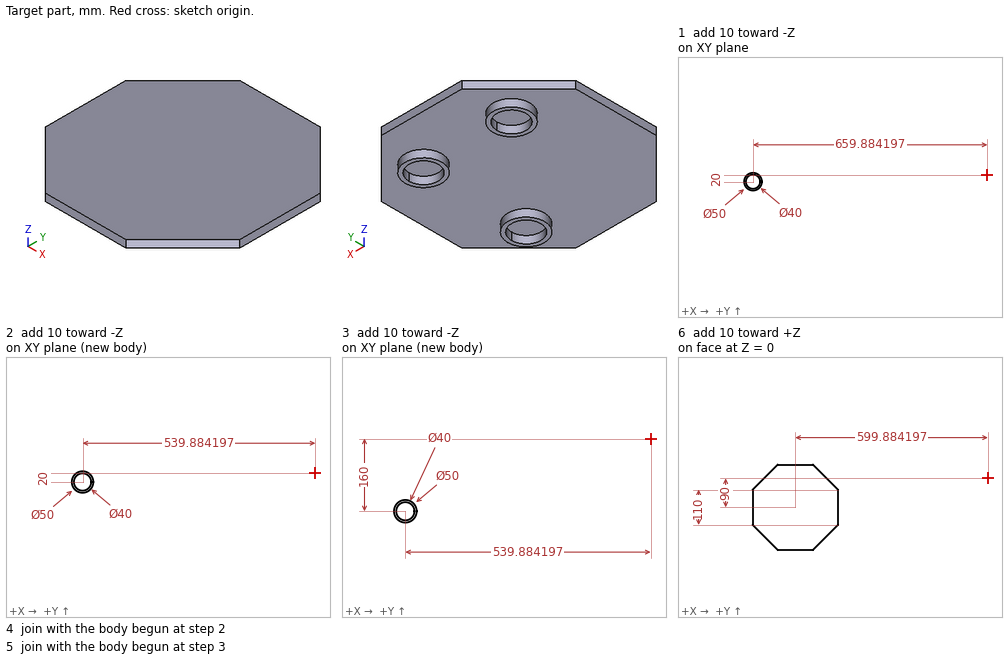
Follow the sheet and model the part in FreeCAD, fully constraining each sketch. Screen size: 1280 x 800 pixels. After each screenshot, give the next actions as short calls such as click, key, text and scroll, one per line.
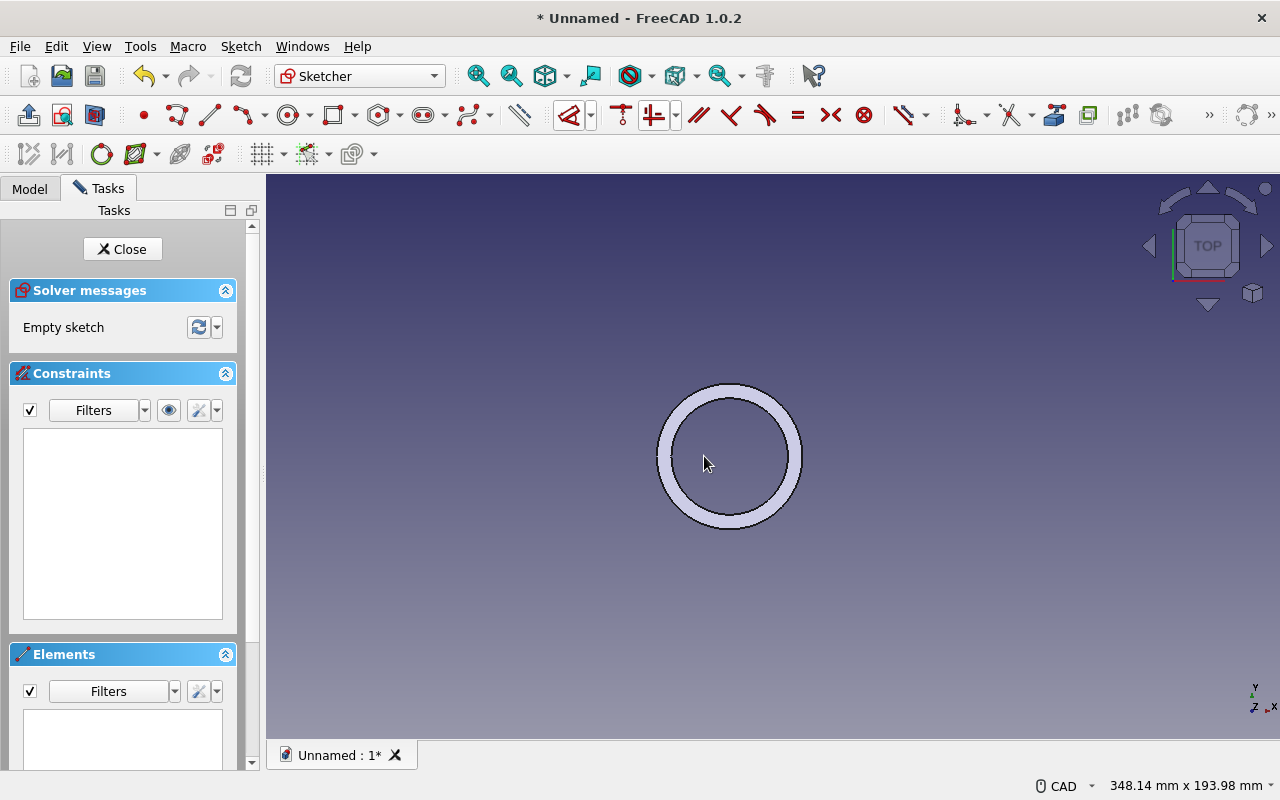
scroll(704, 456, down, 5)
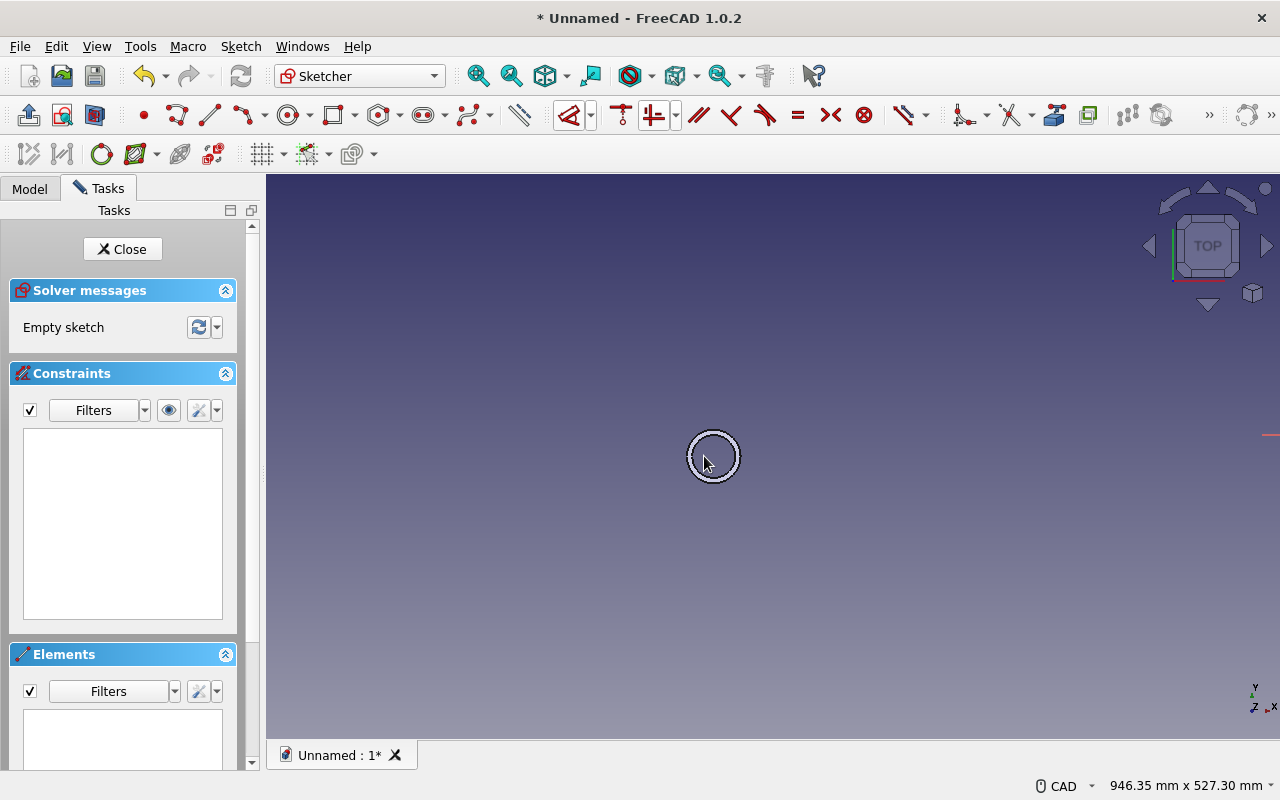
scroll(864, 456, up, 10)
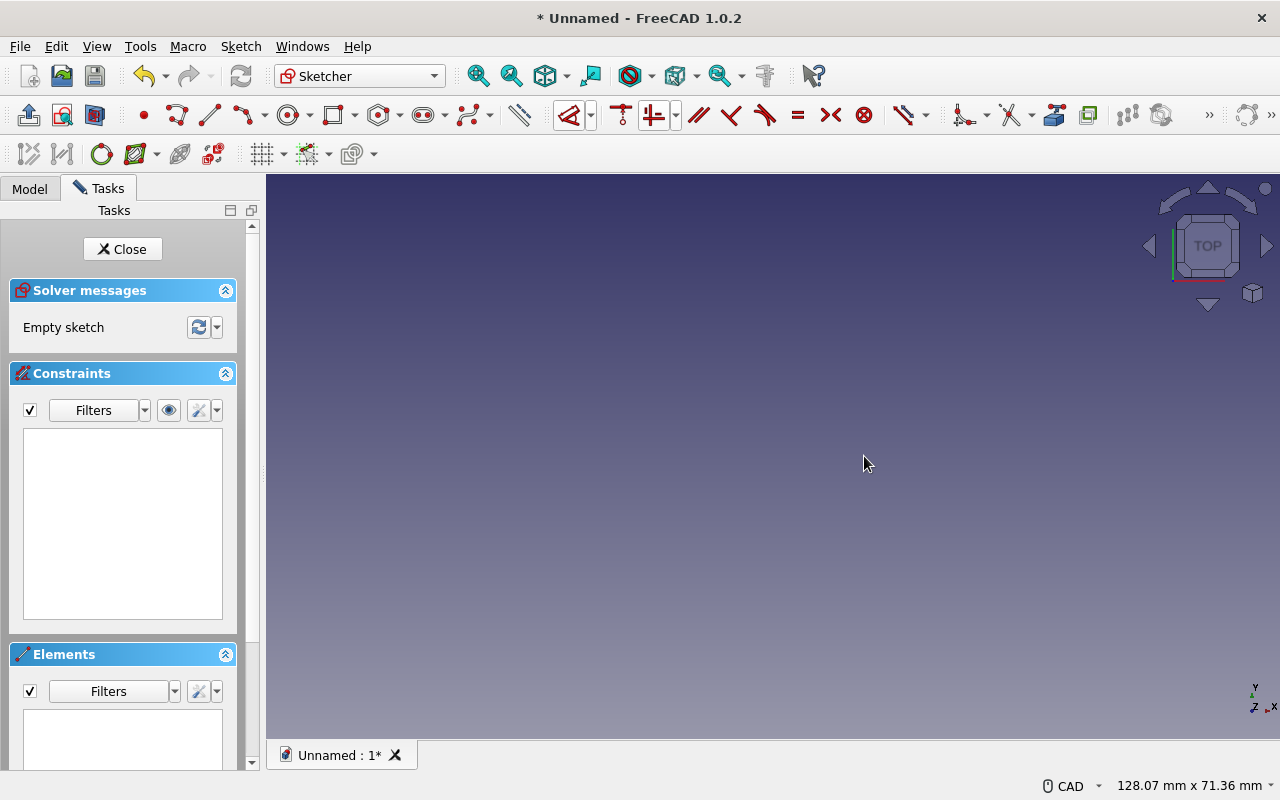
key(g)
key(c)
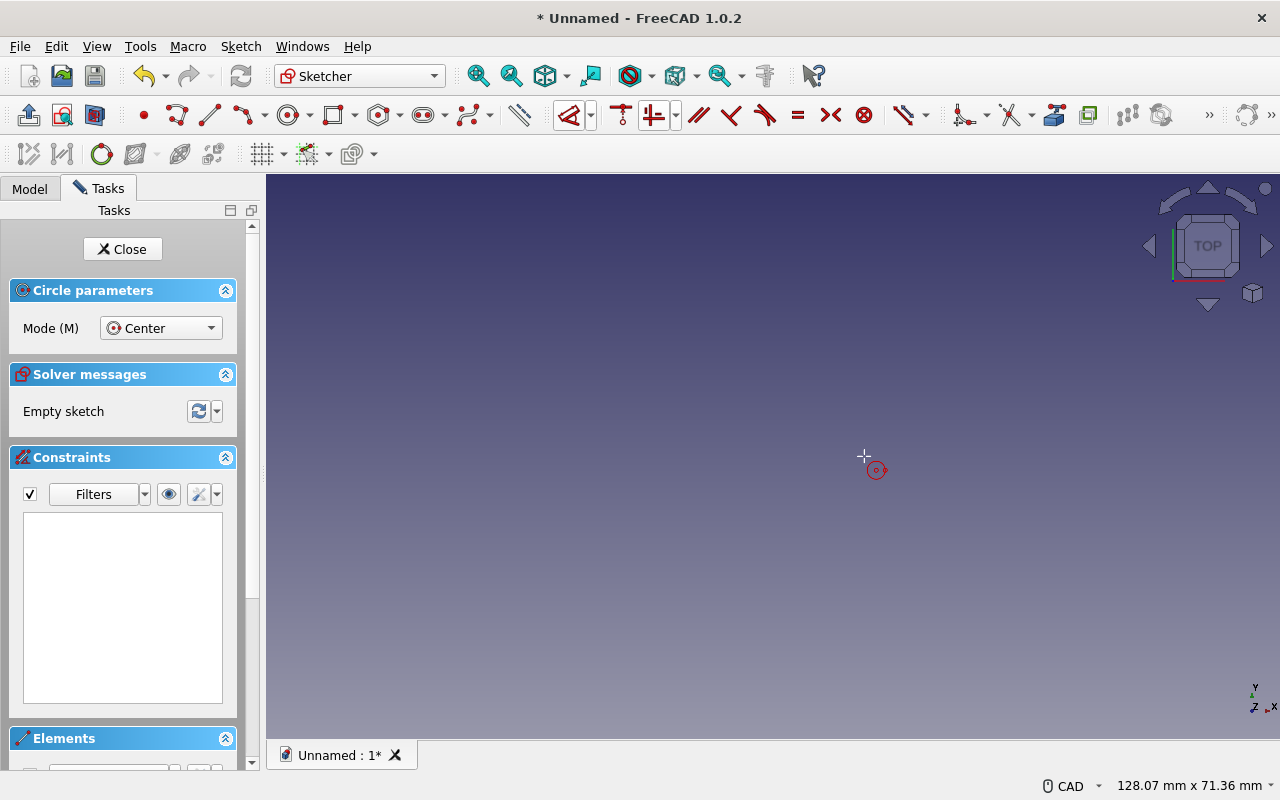
click(700, 456)
move(840, 317)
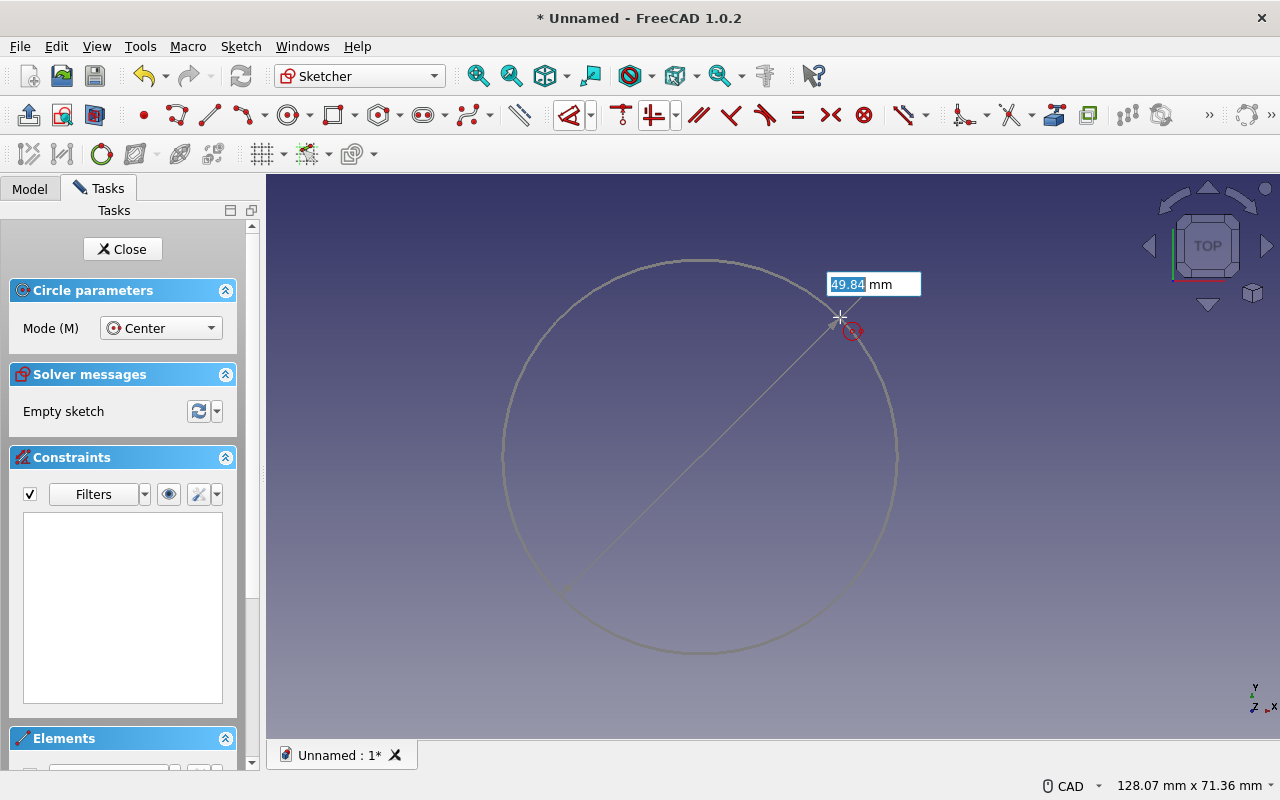
text(50)
key(Return)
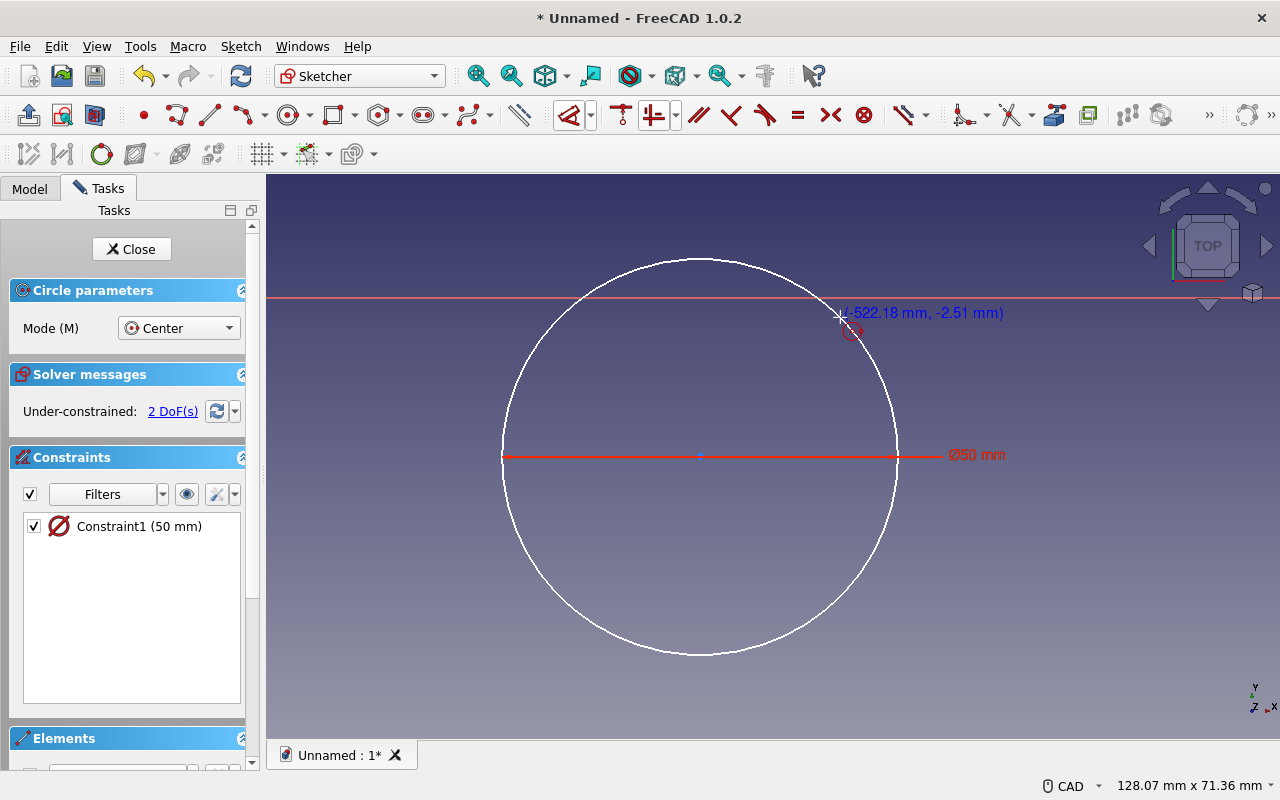
click(700, 457)
move(812, 345)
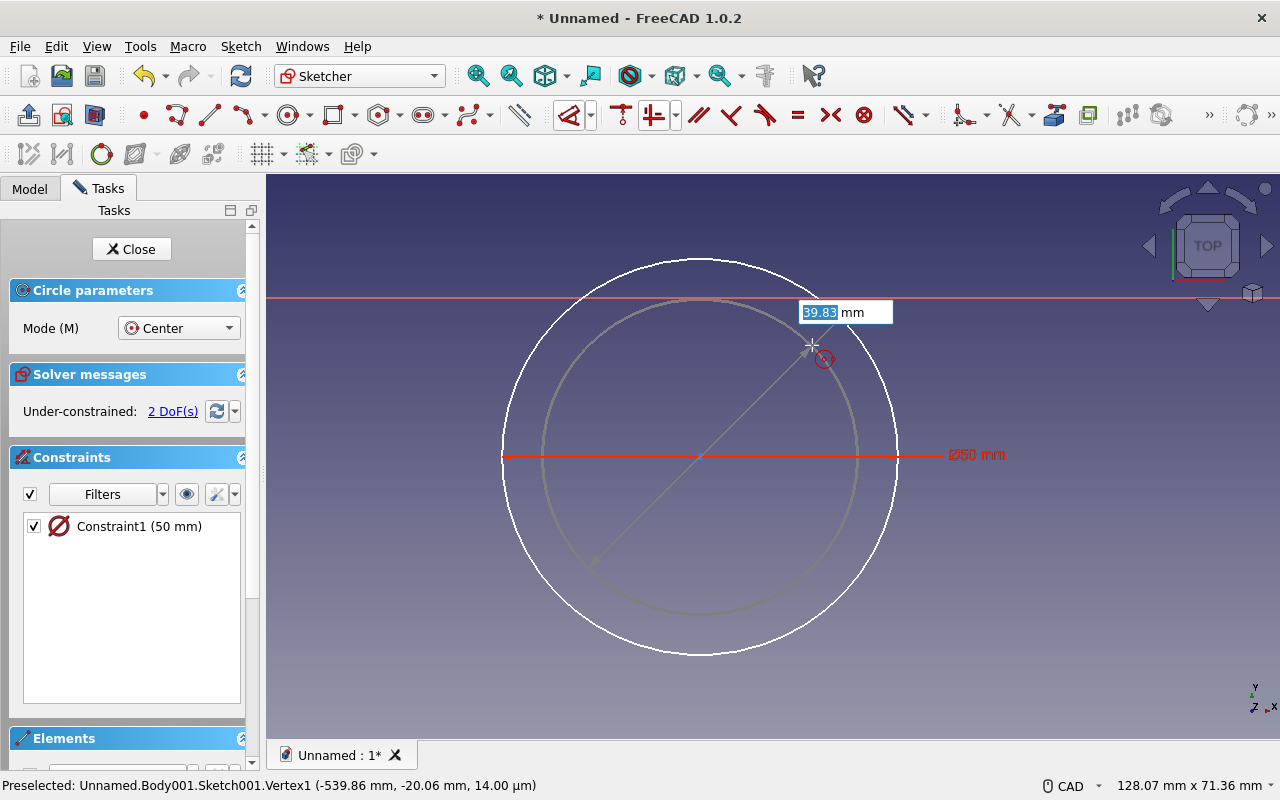
text(40)
key(Return)
key(Escape)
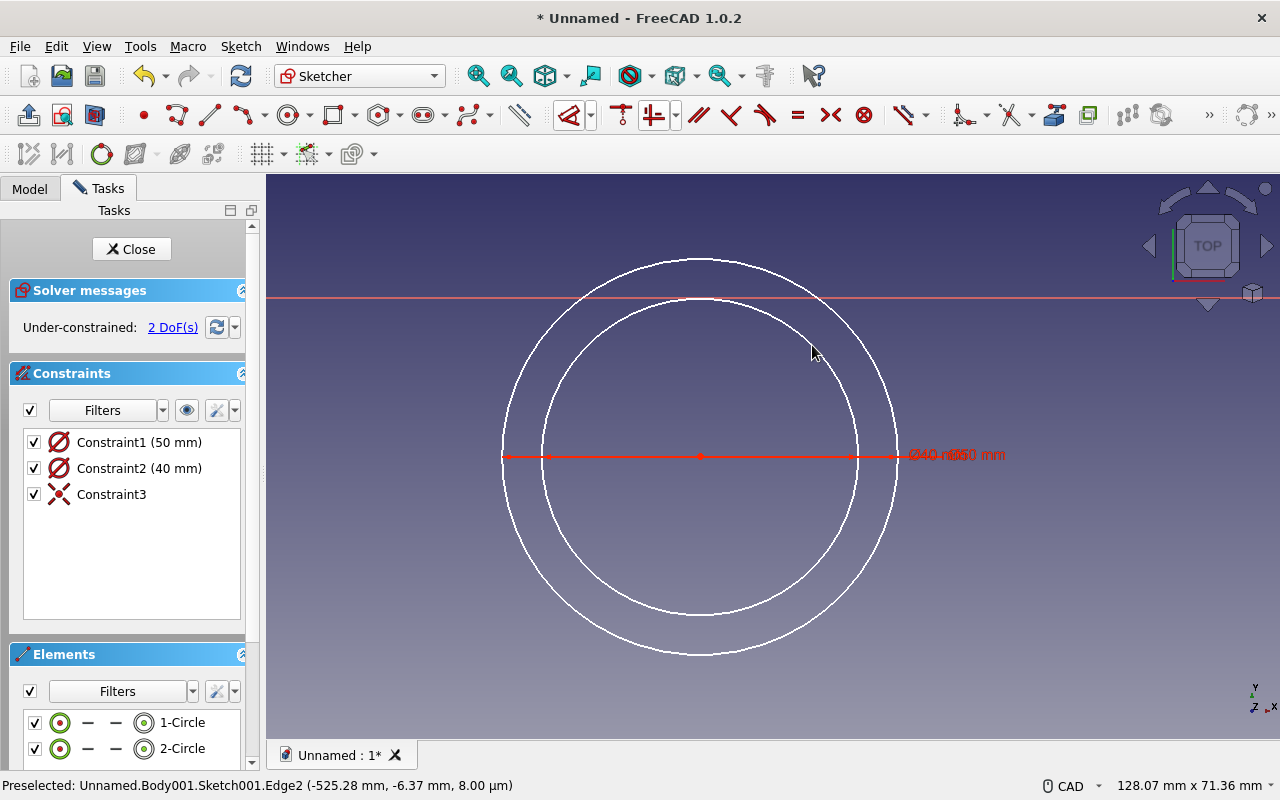
click(568, 116)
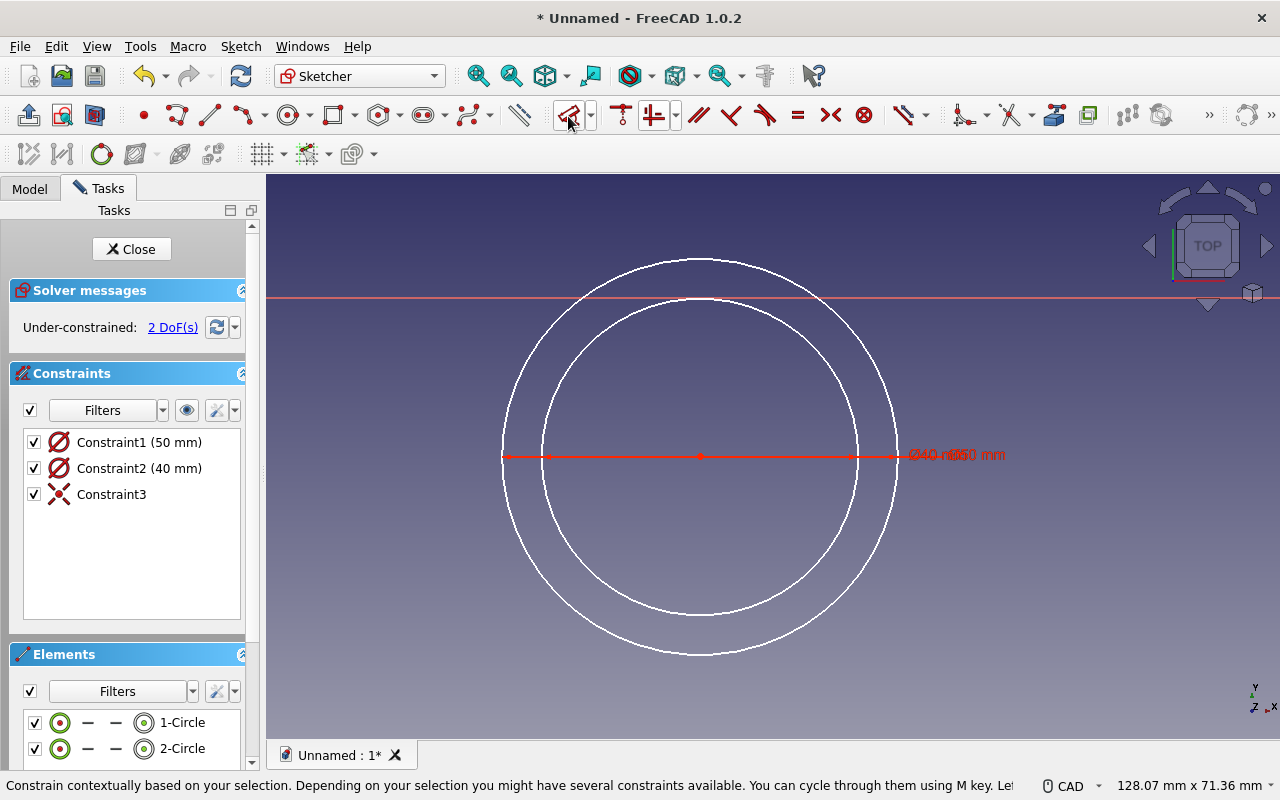
click(700, 457)
click(666, 378)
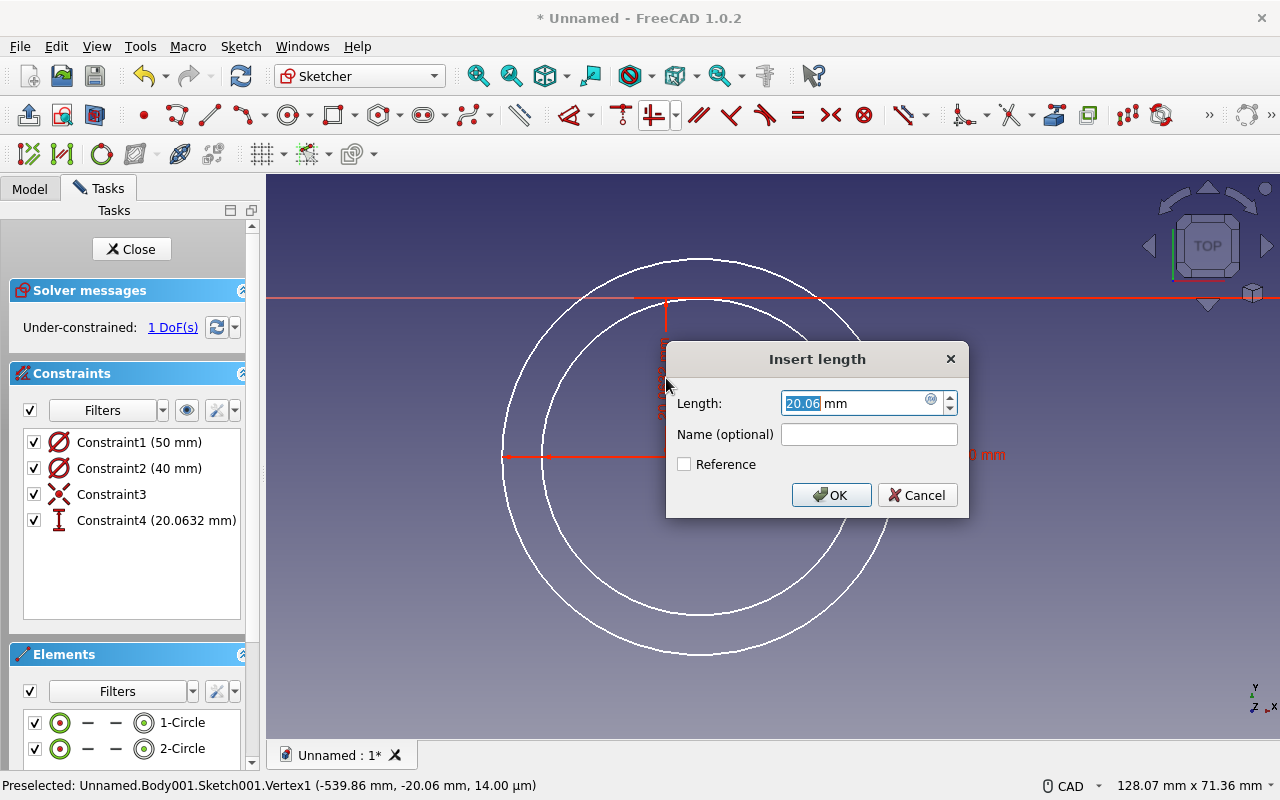
text(20)
key(Return)